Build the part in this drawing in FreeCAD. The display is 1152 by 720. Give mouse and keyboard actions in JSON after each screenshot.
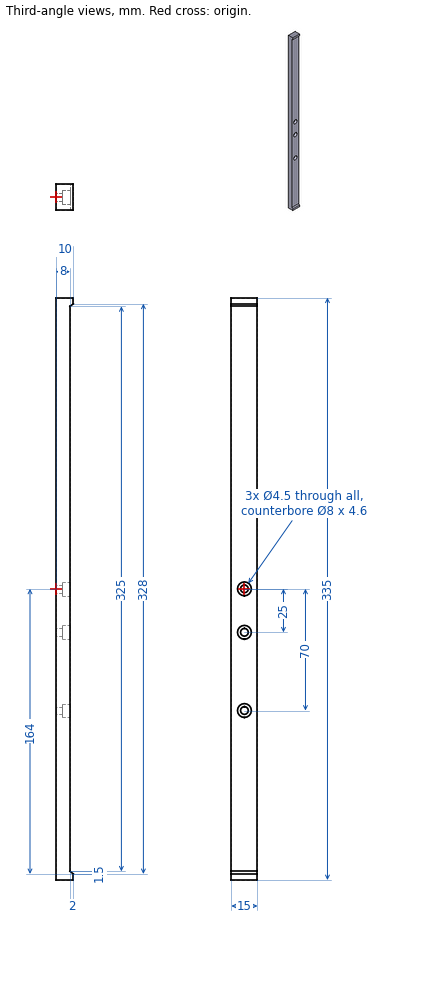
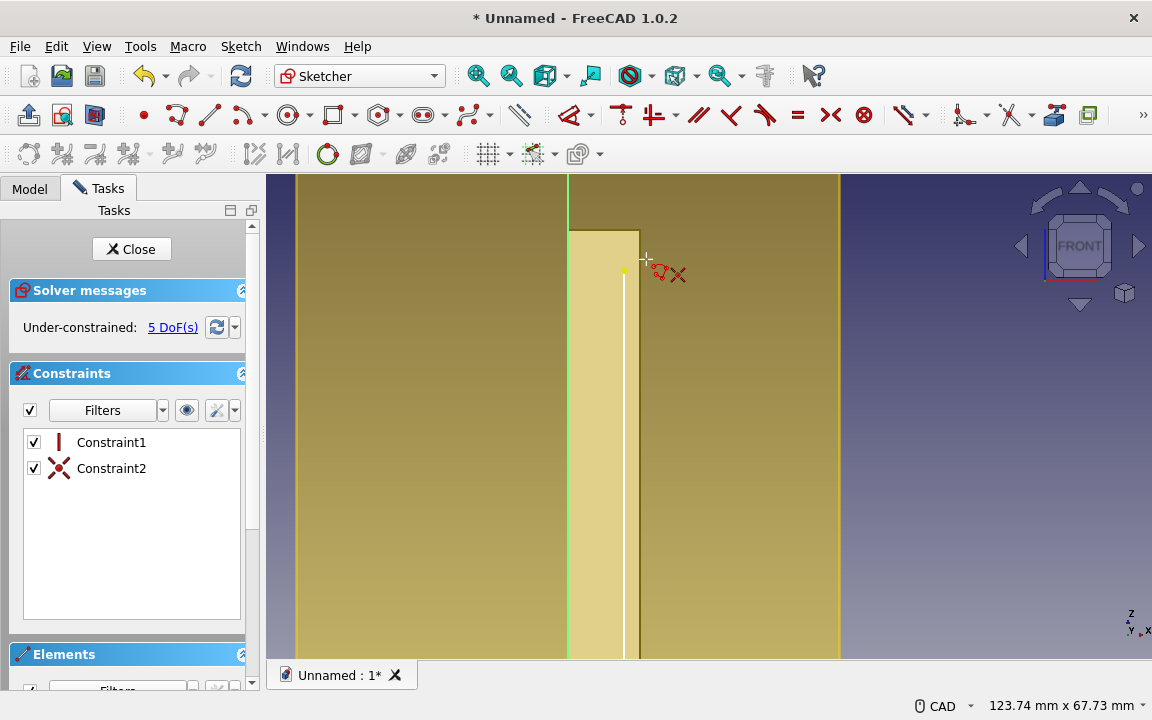
{"action": "left_click", "coordinate": [640, 255]}
{"action": "left_click", "coordinate": [624, 270]}
{"action": "key", "text": "Escape"}
{"action": "key", "text": "Escape"}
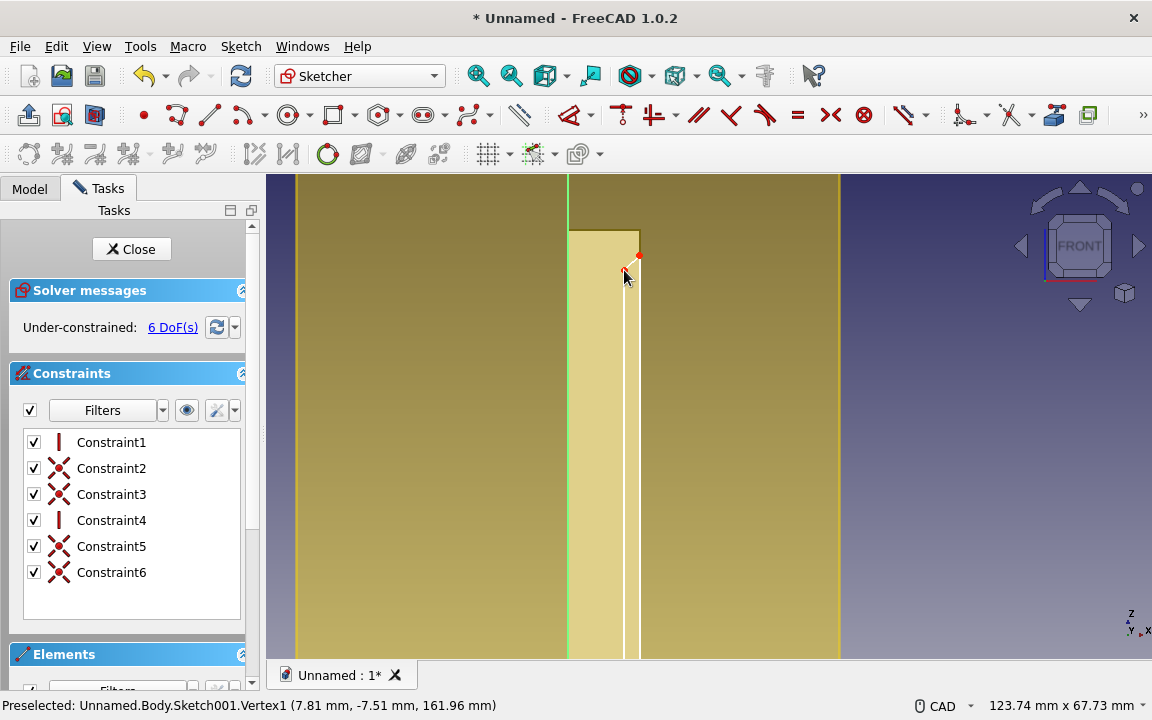
{"action": "left_click", "coordinate": [624, 270]}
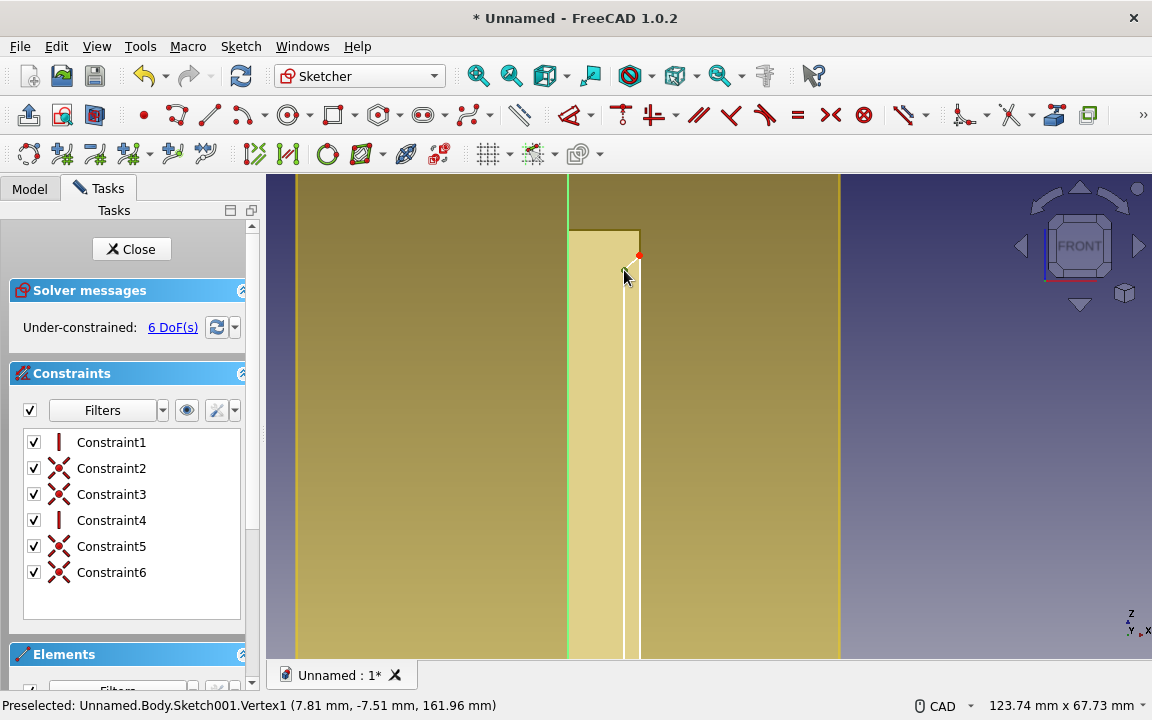
{"action": "left_click", "coordinate": [590, 116]}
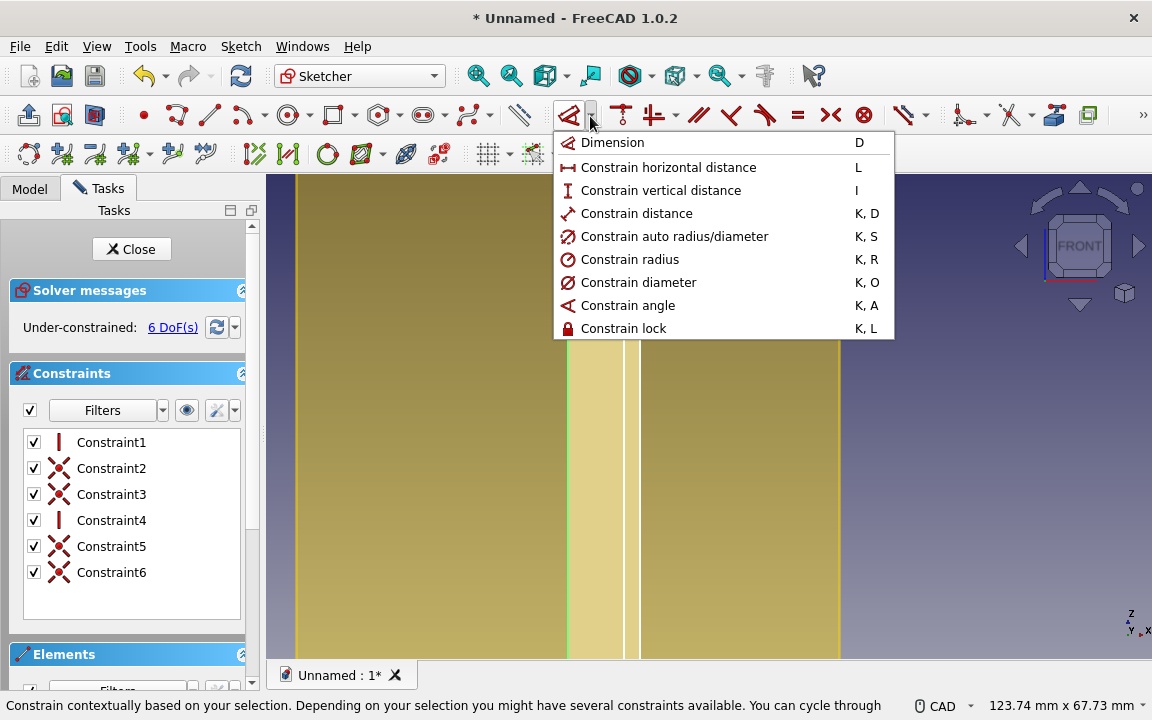
{"action": "left_click", "coordinate": [724, 168]}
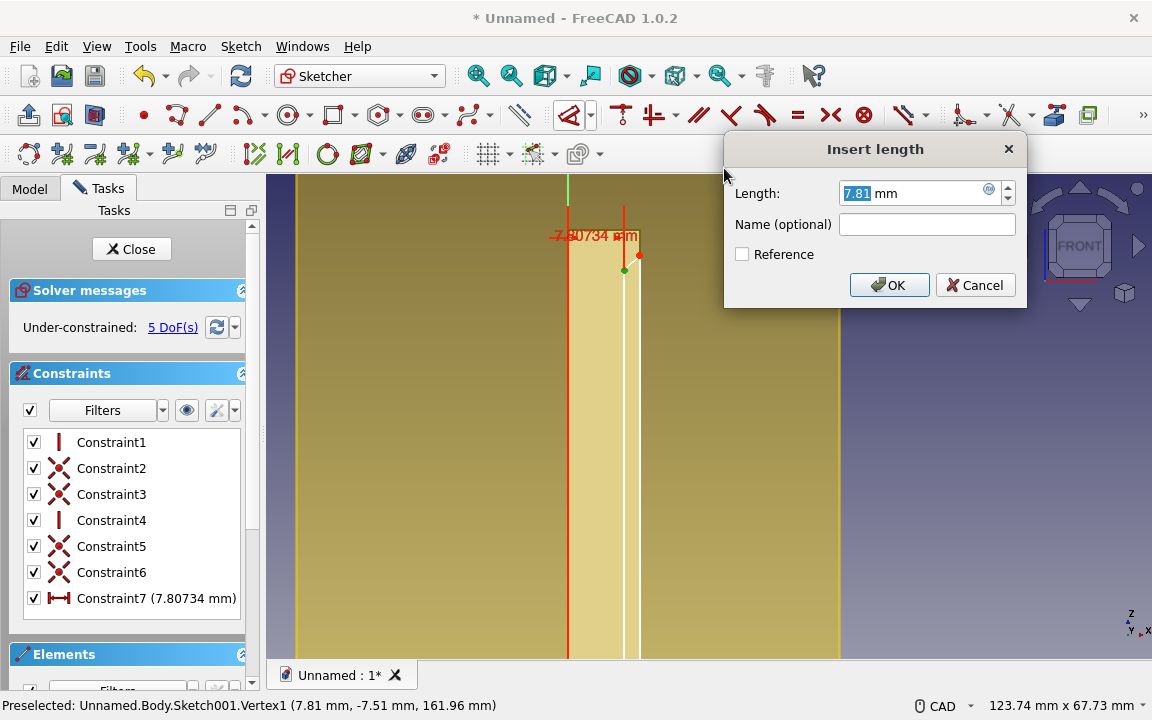
{"action": "type", "text": "8"}
{"action": "key", "text": "Return"}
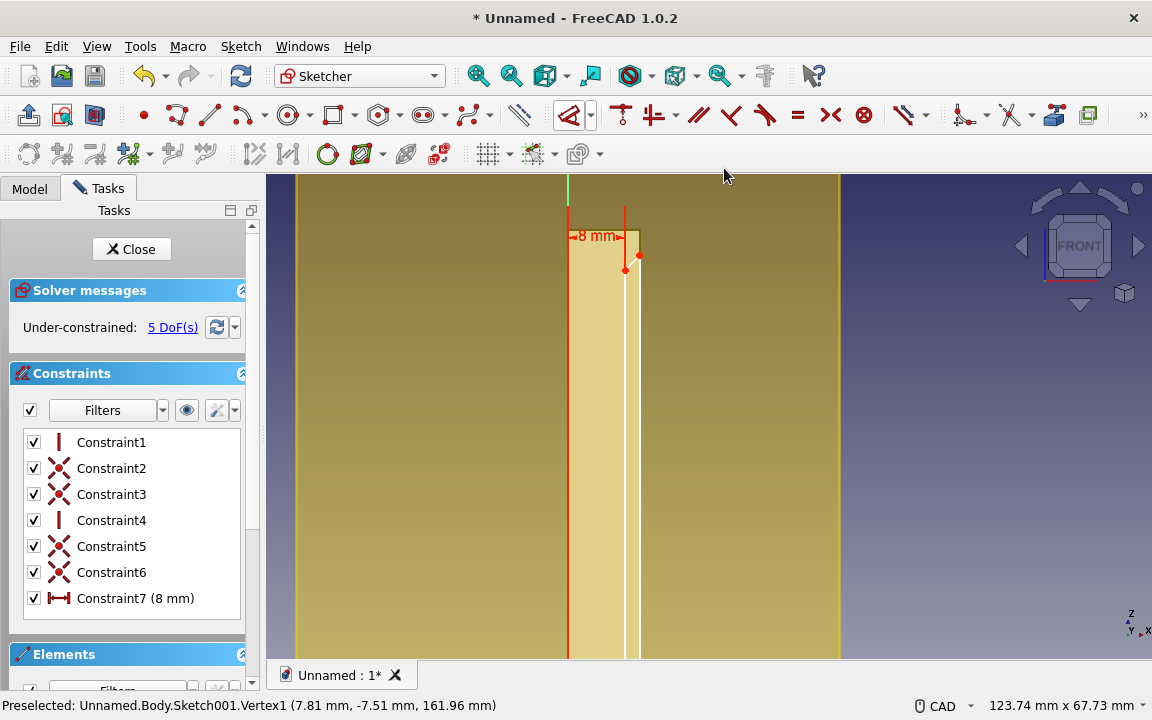
{"action": "scroll", "coordinate": [646, 258], "scroll_direction": "down", "scroll_amount": 10}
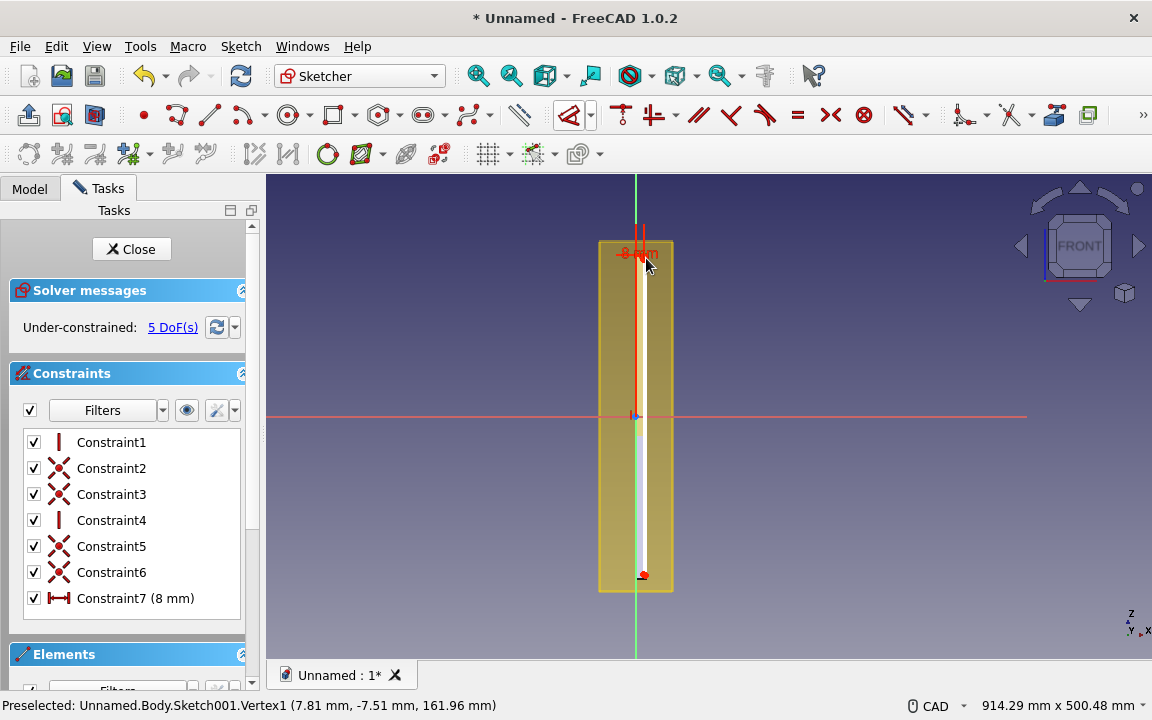
{"action": "scroll", "coordinate": [645, 575], "scroll_direction": "up", "scroll_amount": 16}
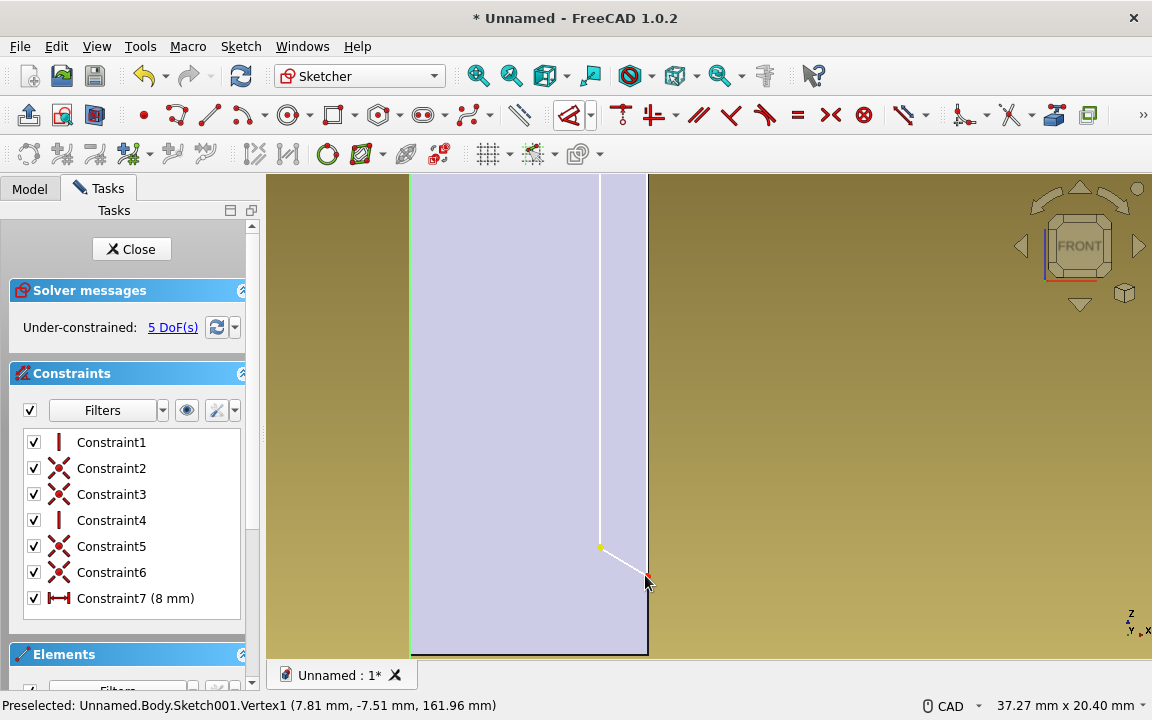
{"action": "left_click", "coordinate": [624, 562]}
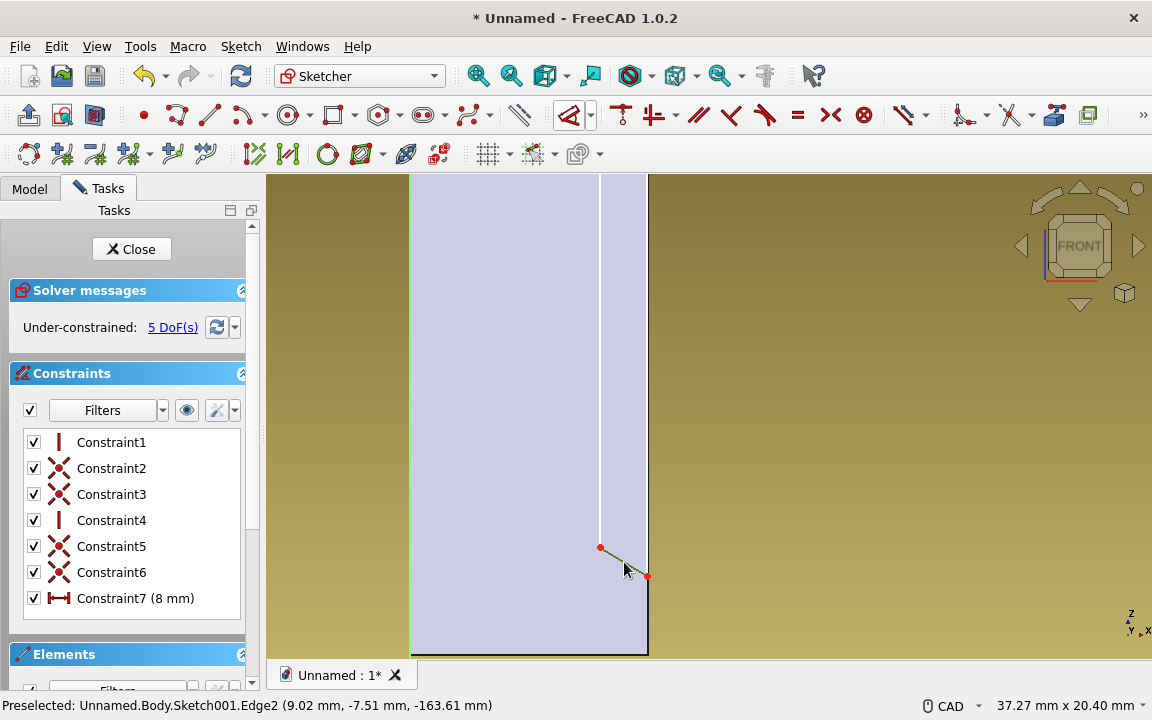
{"action": "left_click", "coordinate": [590, 116]}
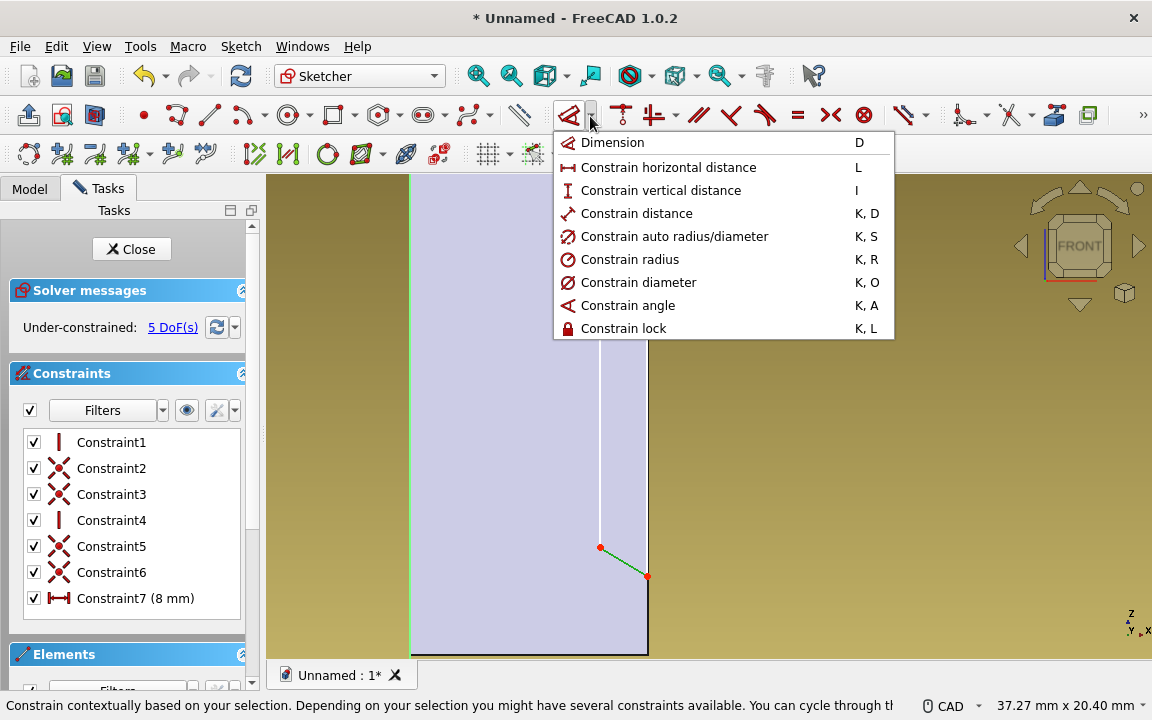
{"action": "left_click", "coordinate": [724, 168]}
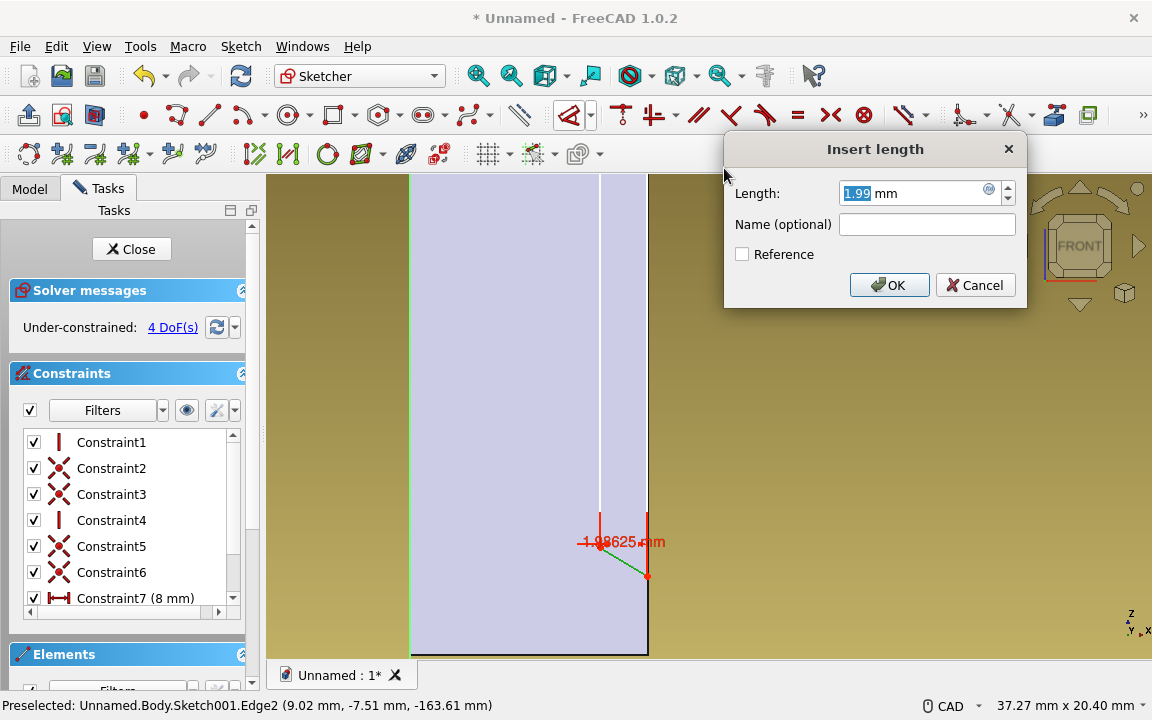
{"action": "type", "text": "2"}
{"action": "key", "text": "Return"}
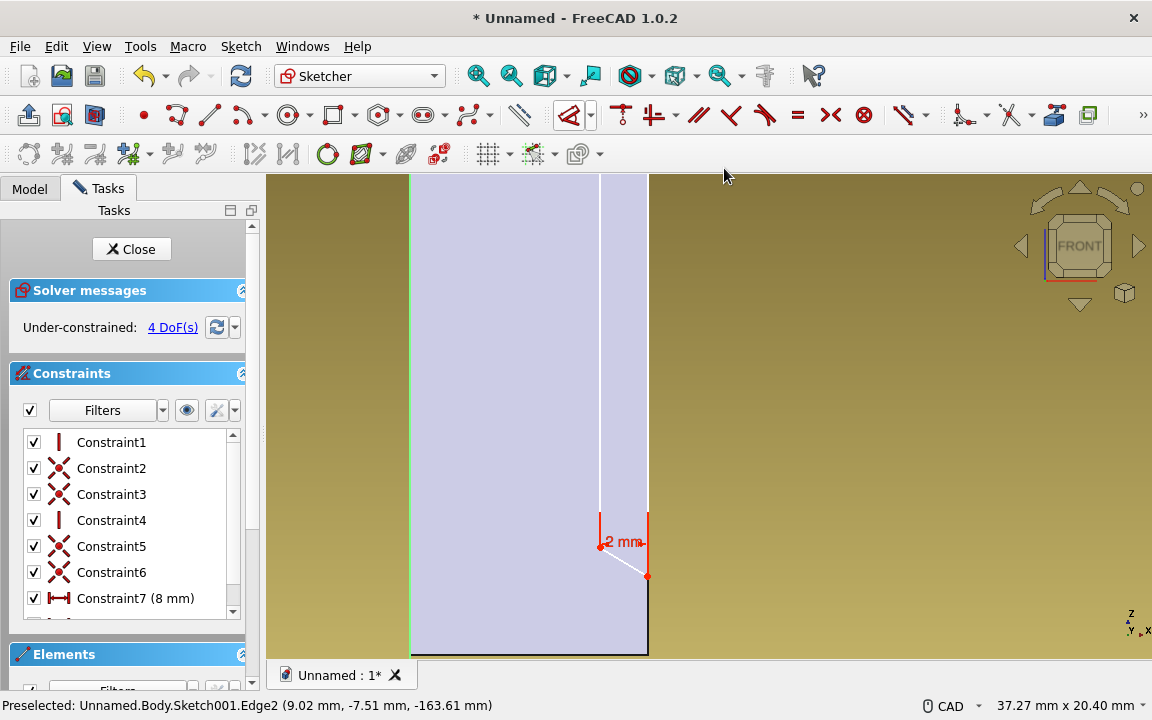
{"action": "scroll", "coordinate": [645, 576], "scroll_direction": "down", "scroll_amount": 16}